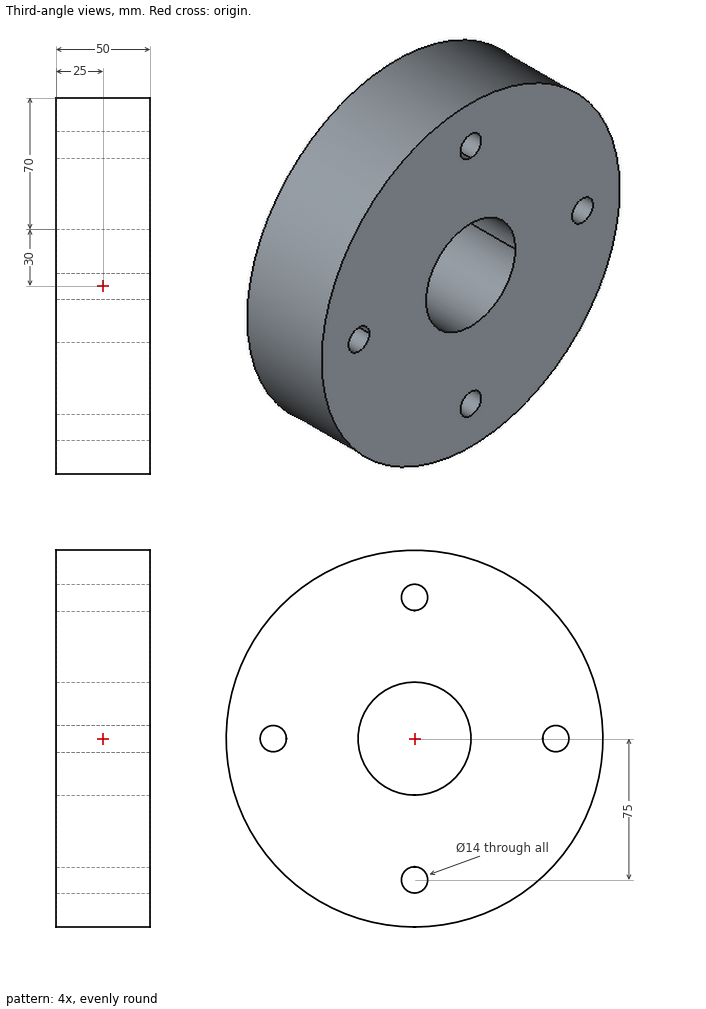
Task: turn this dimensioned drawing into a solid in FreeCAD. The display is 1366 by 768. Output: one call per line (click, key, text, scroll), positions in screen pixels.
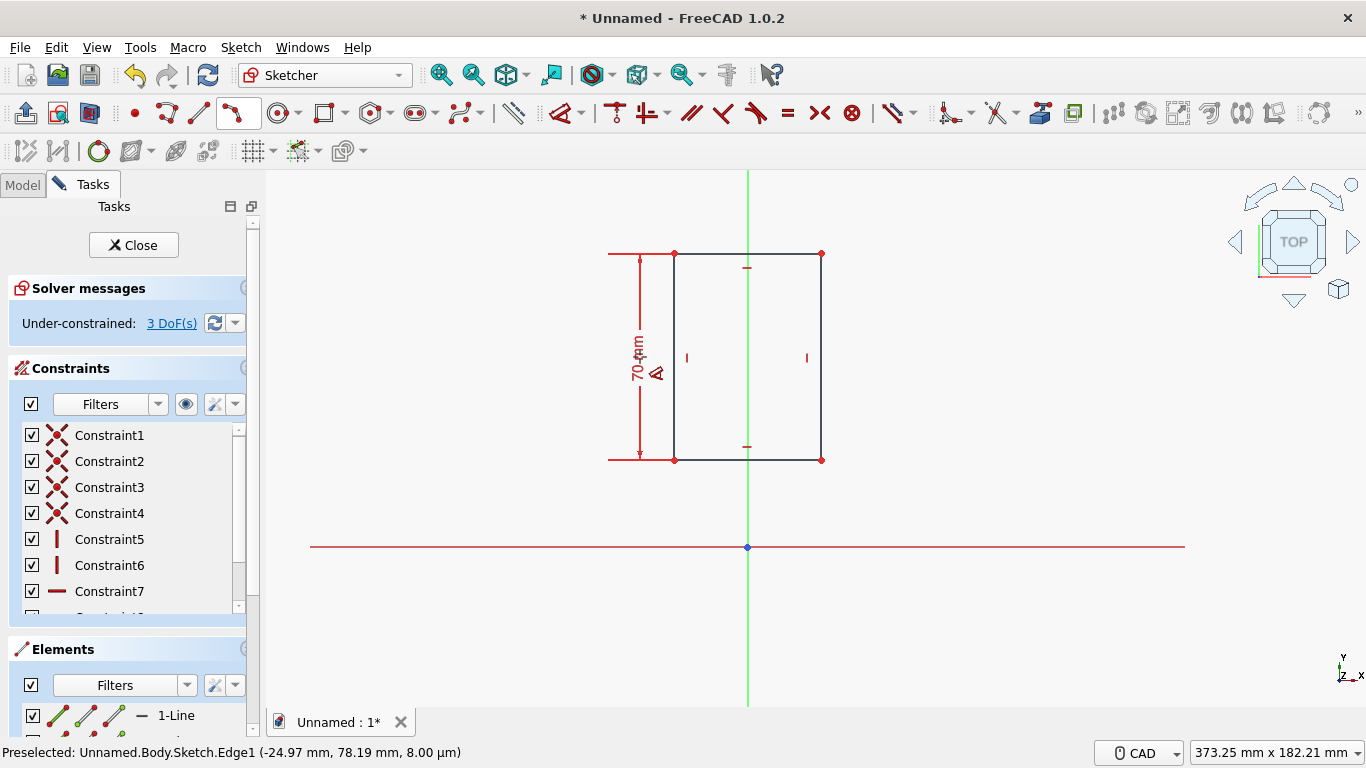
click(718, 460)
click(714, 494)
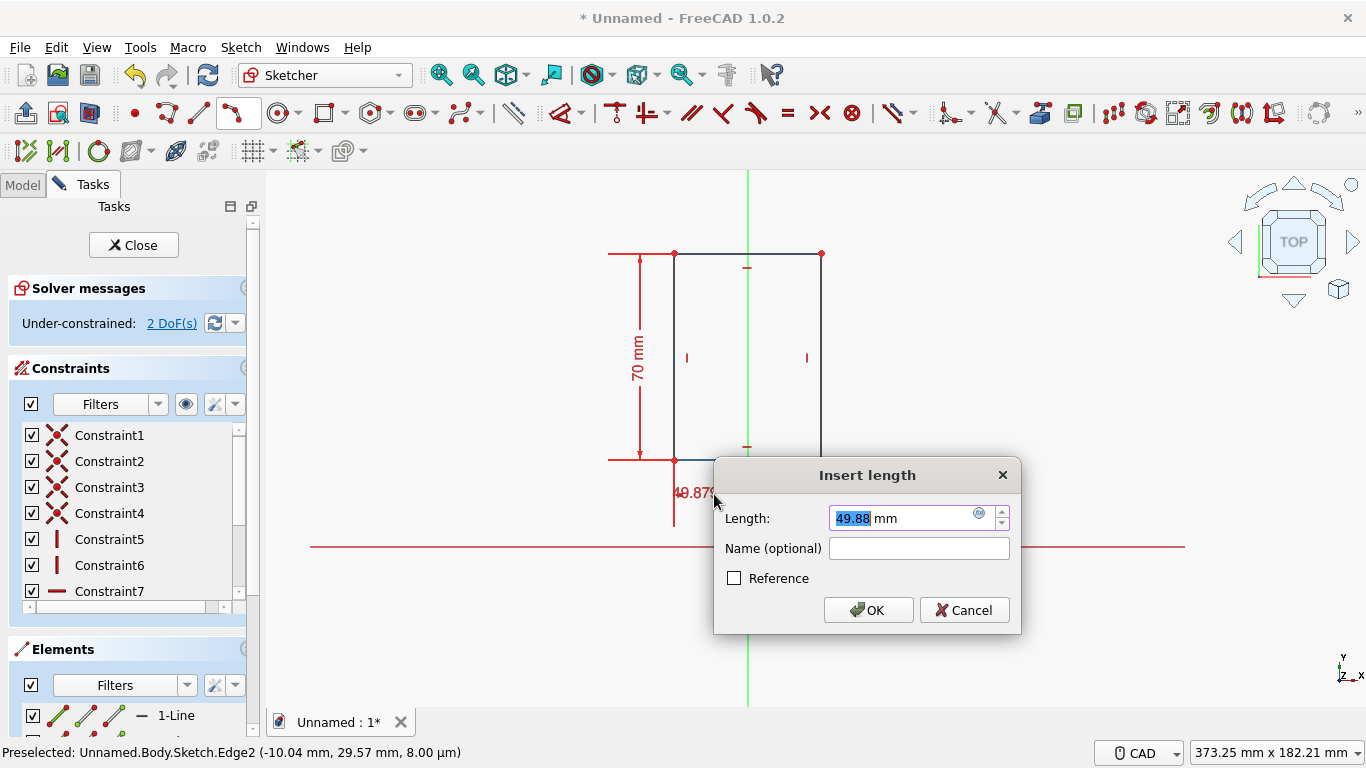
text(50)
key(Return)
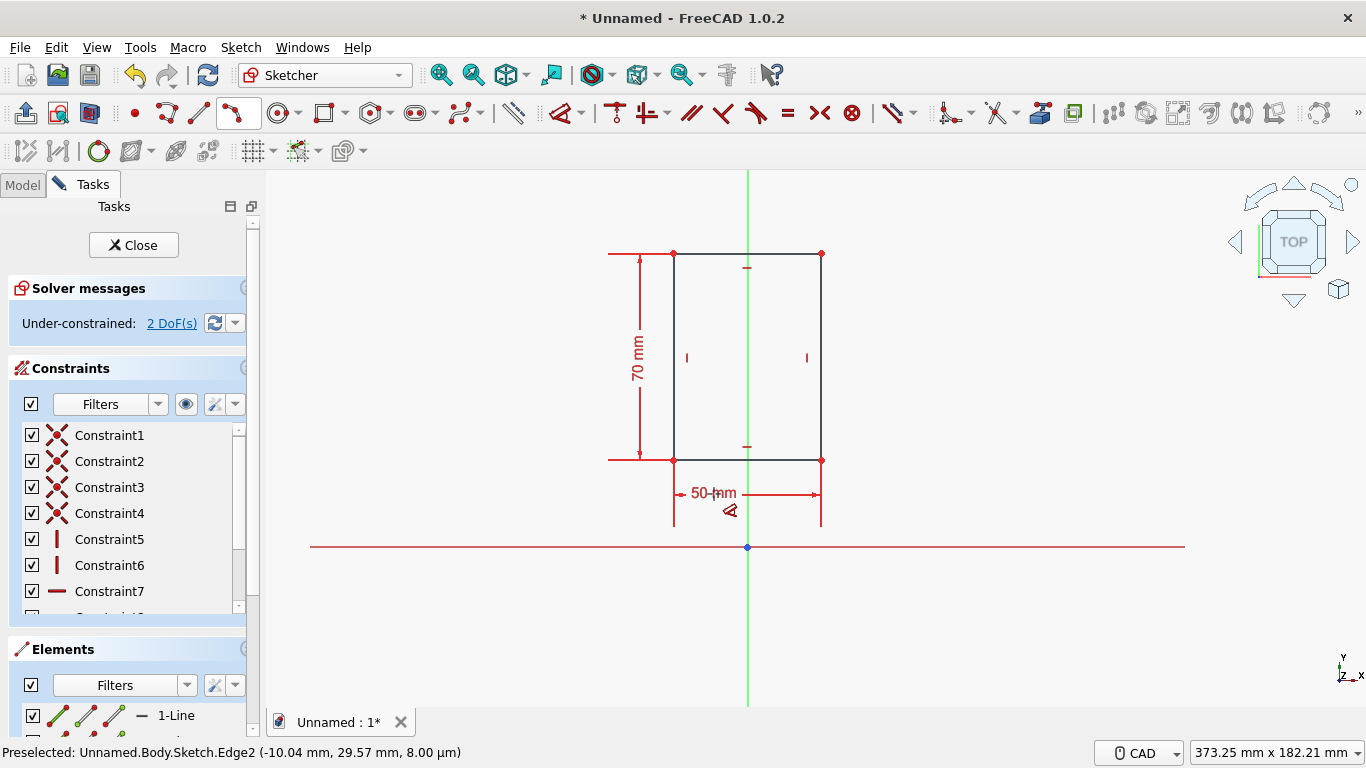
click(674, 254)
click(711, 581)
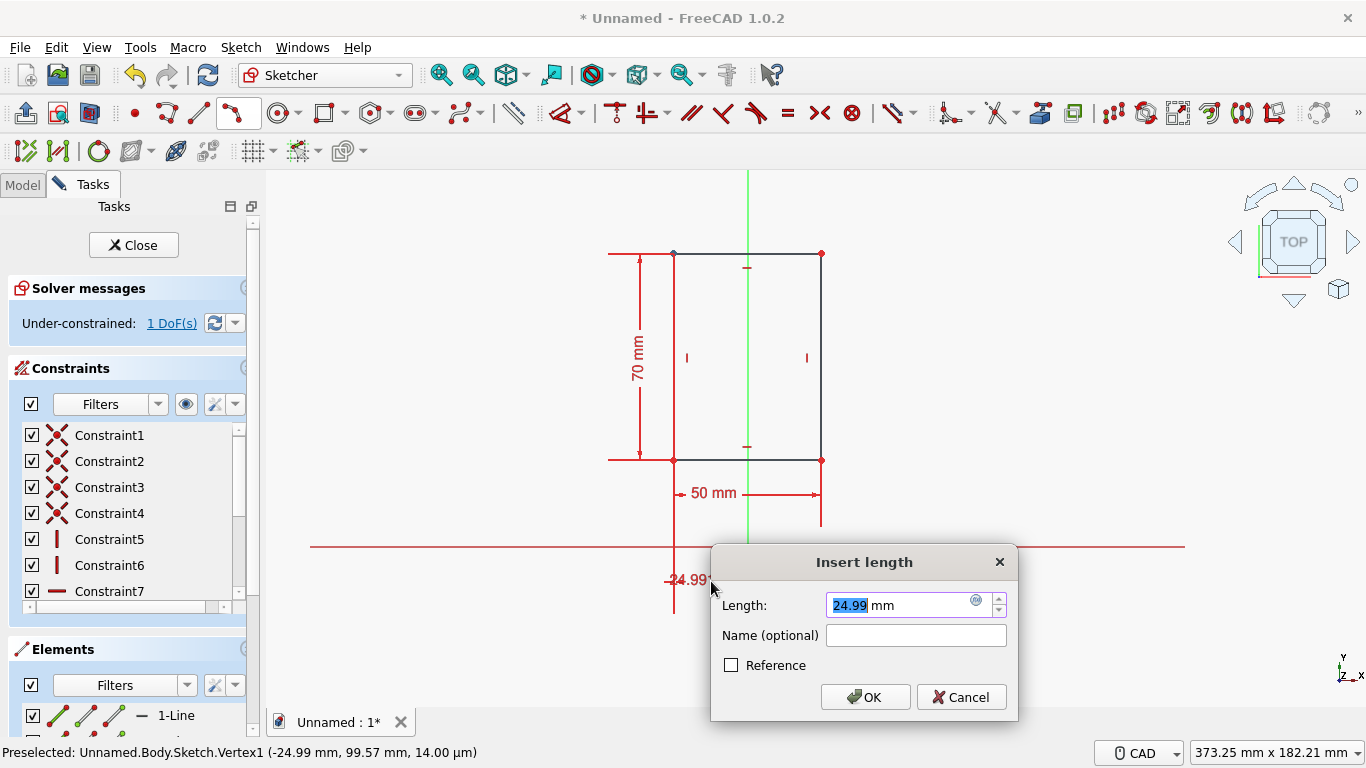
text(25)
key(Return)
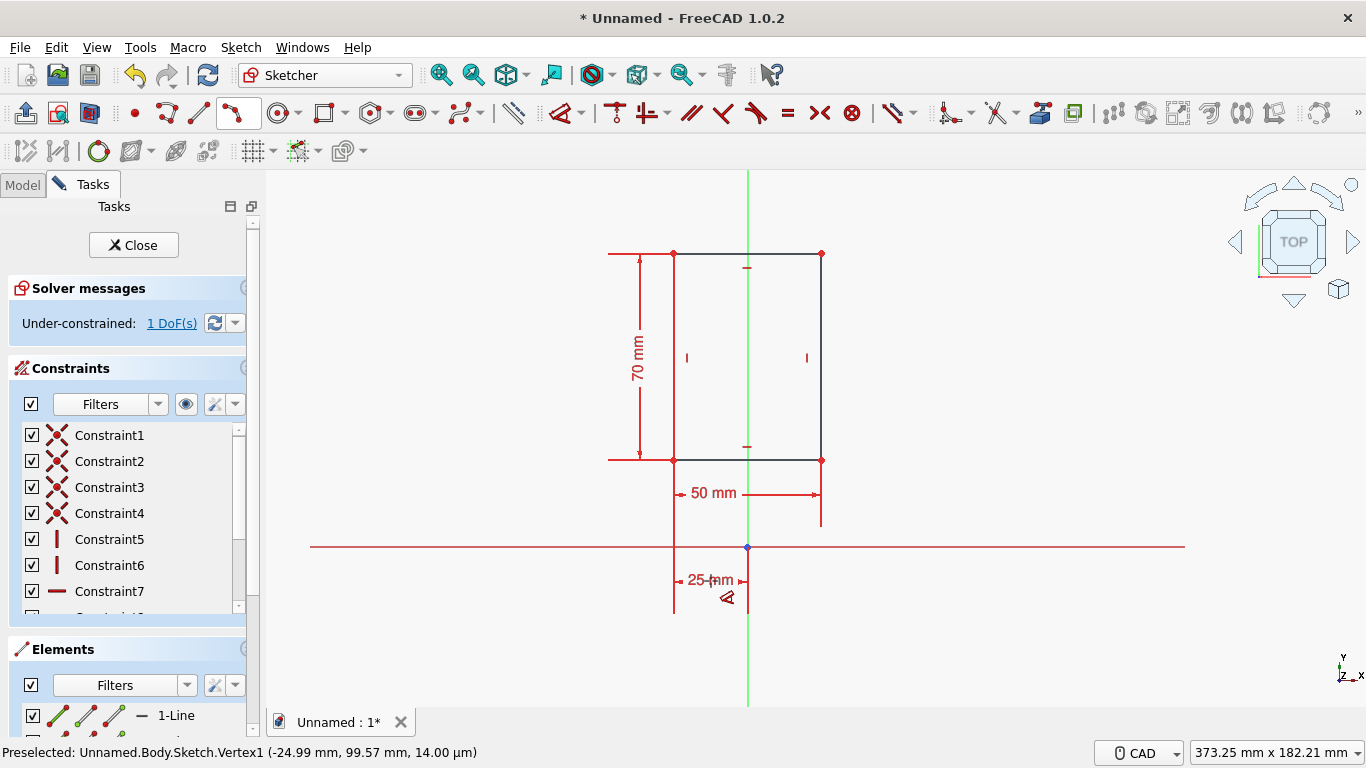
click(674, 460)
click(640, 504)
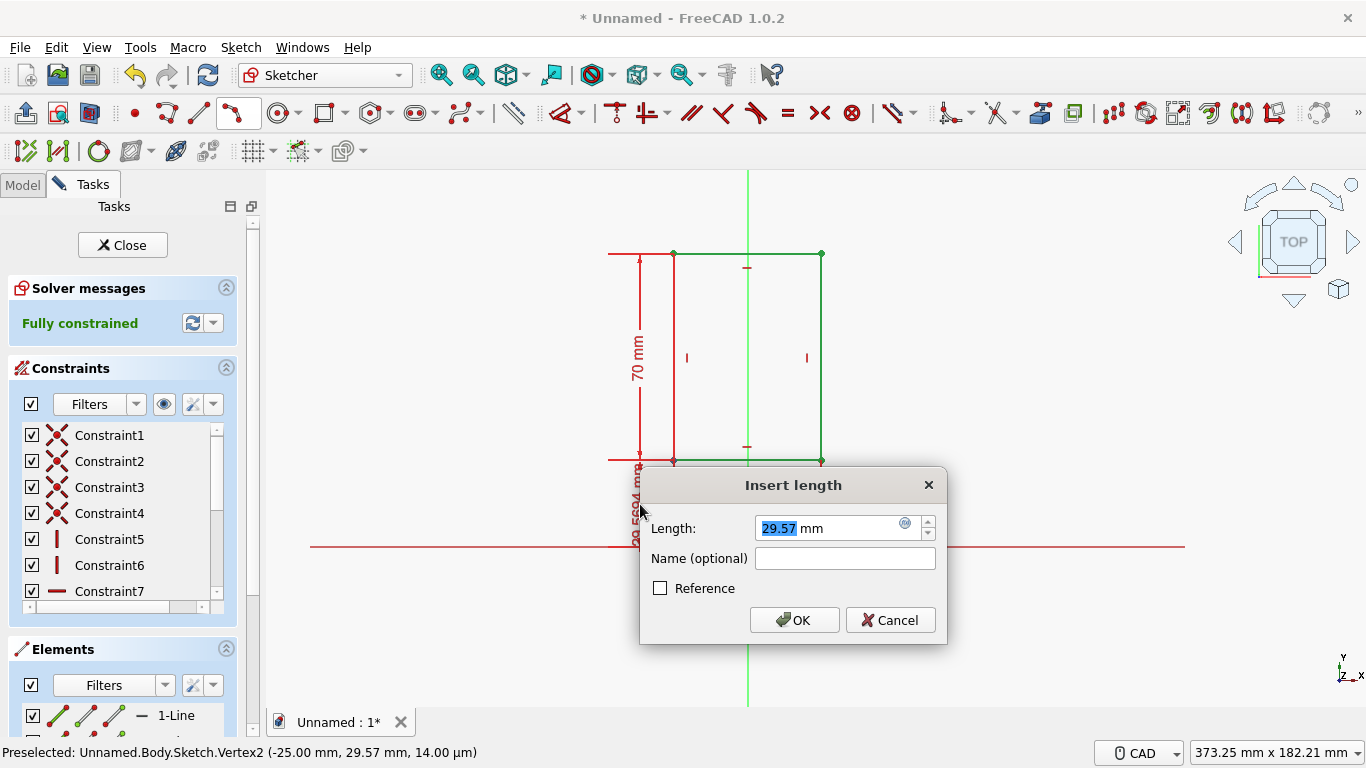
text(30)
key(Return)
key(Escape)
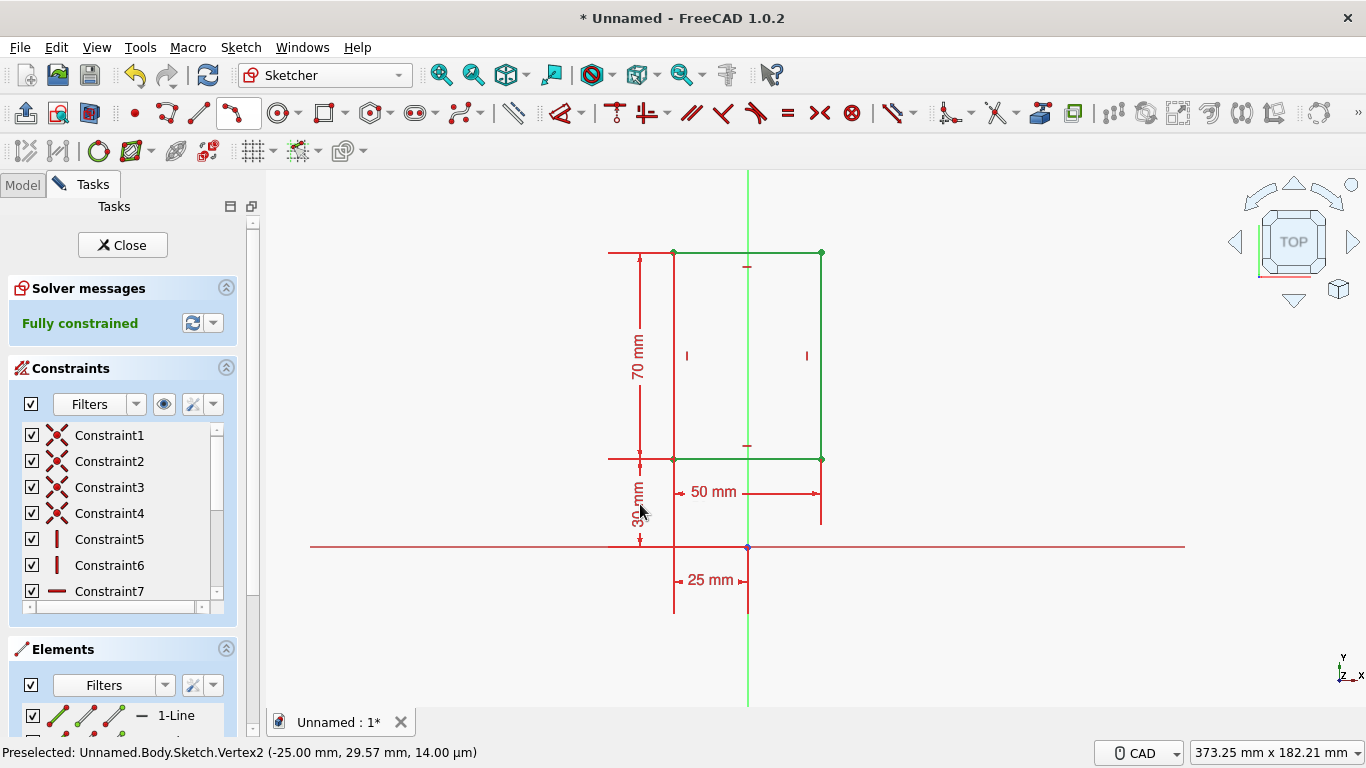
click(123, 245)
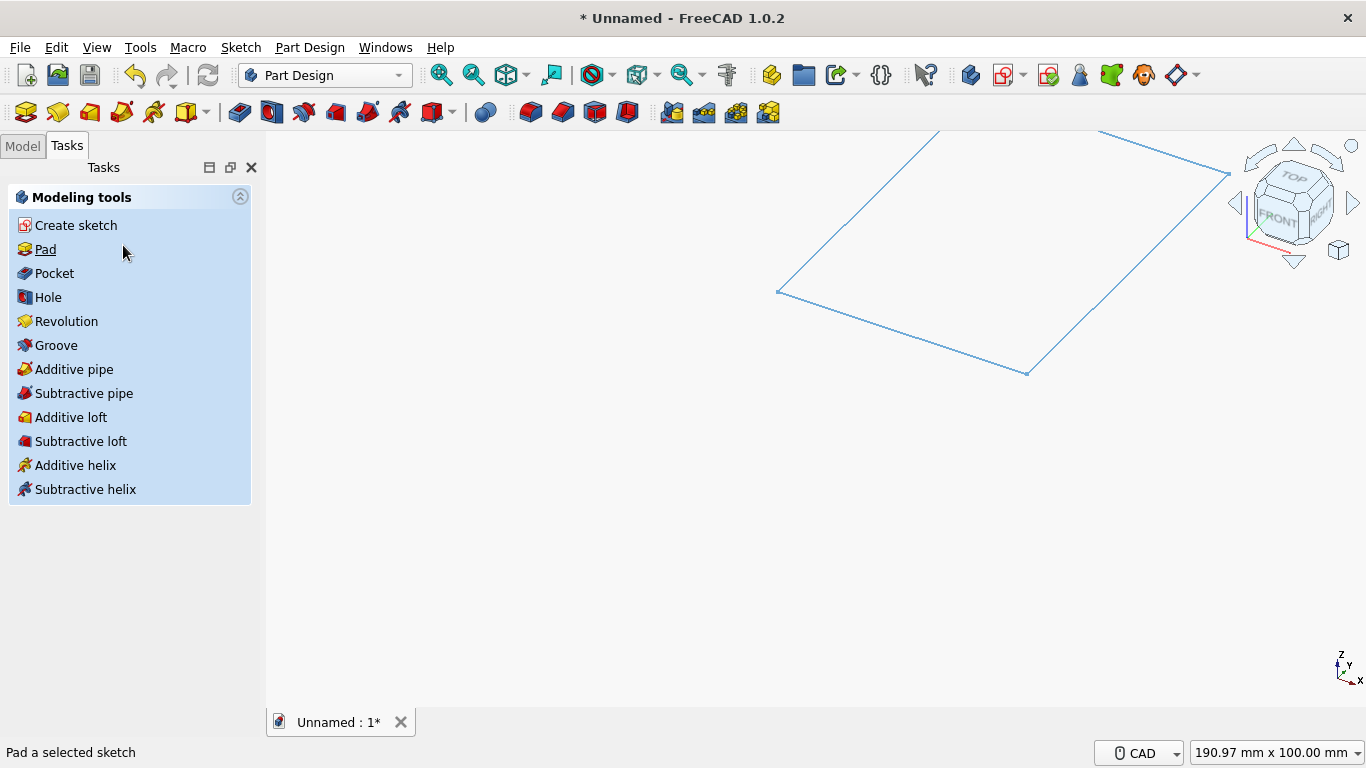
click(58, 112)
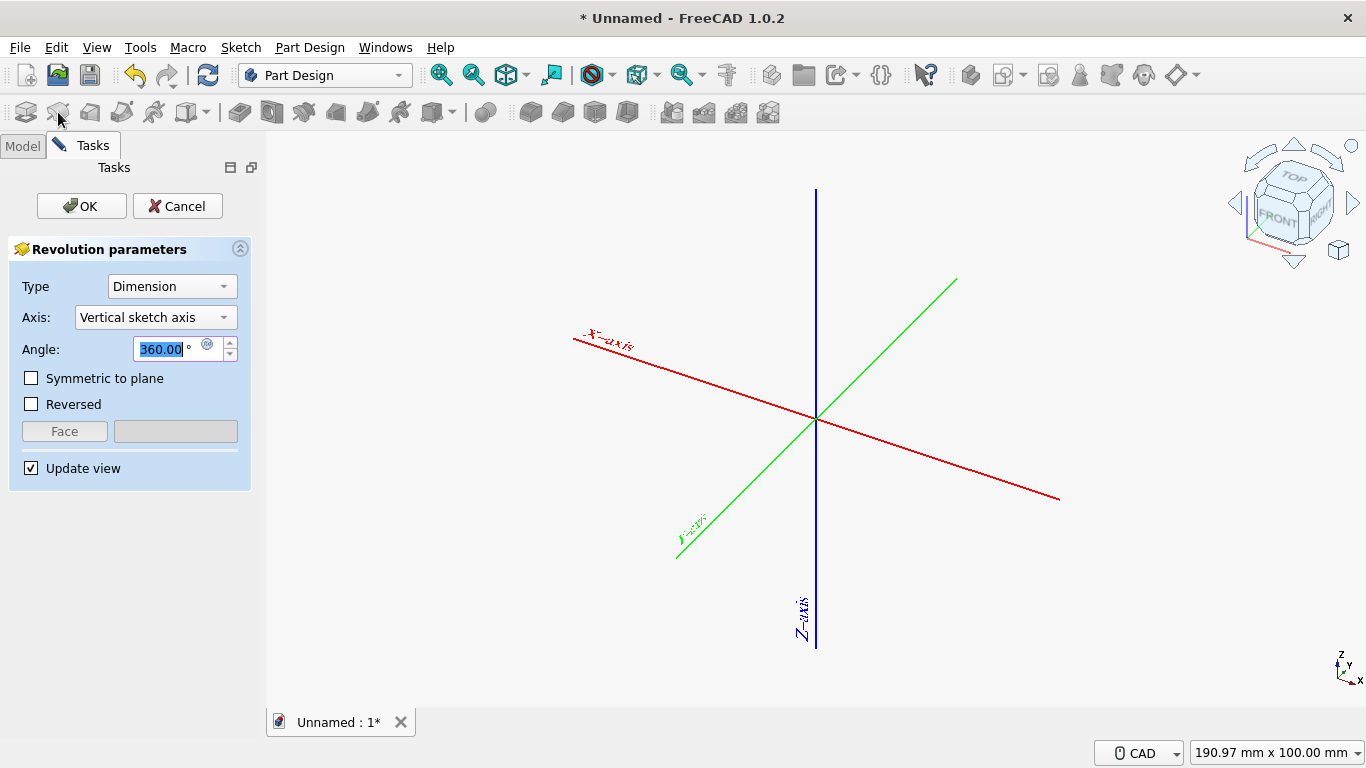
click(156, 318)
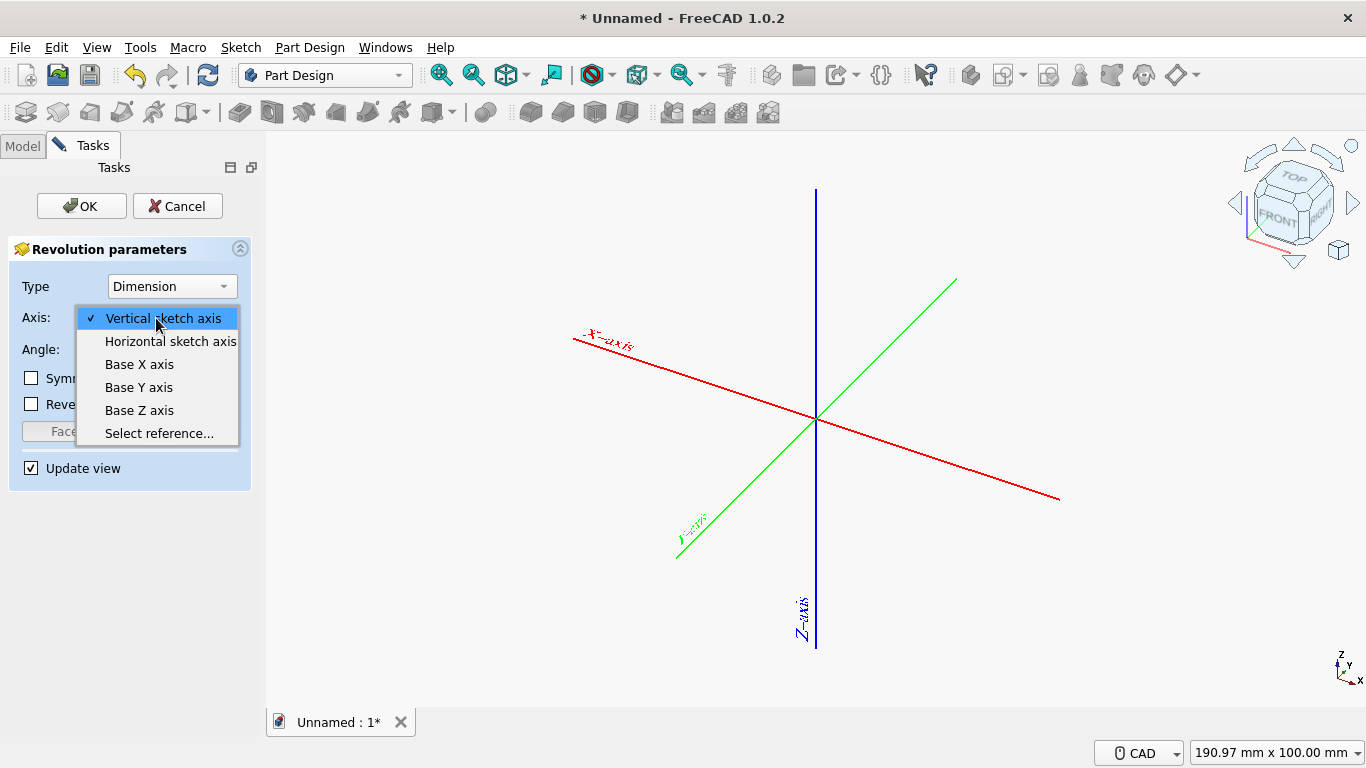
click(156, 342)